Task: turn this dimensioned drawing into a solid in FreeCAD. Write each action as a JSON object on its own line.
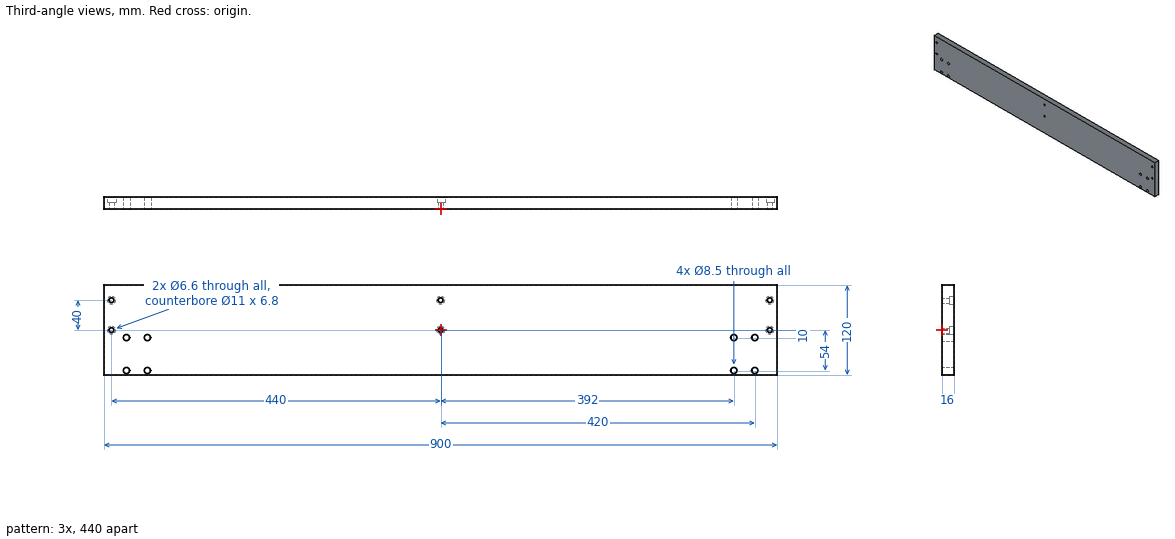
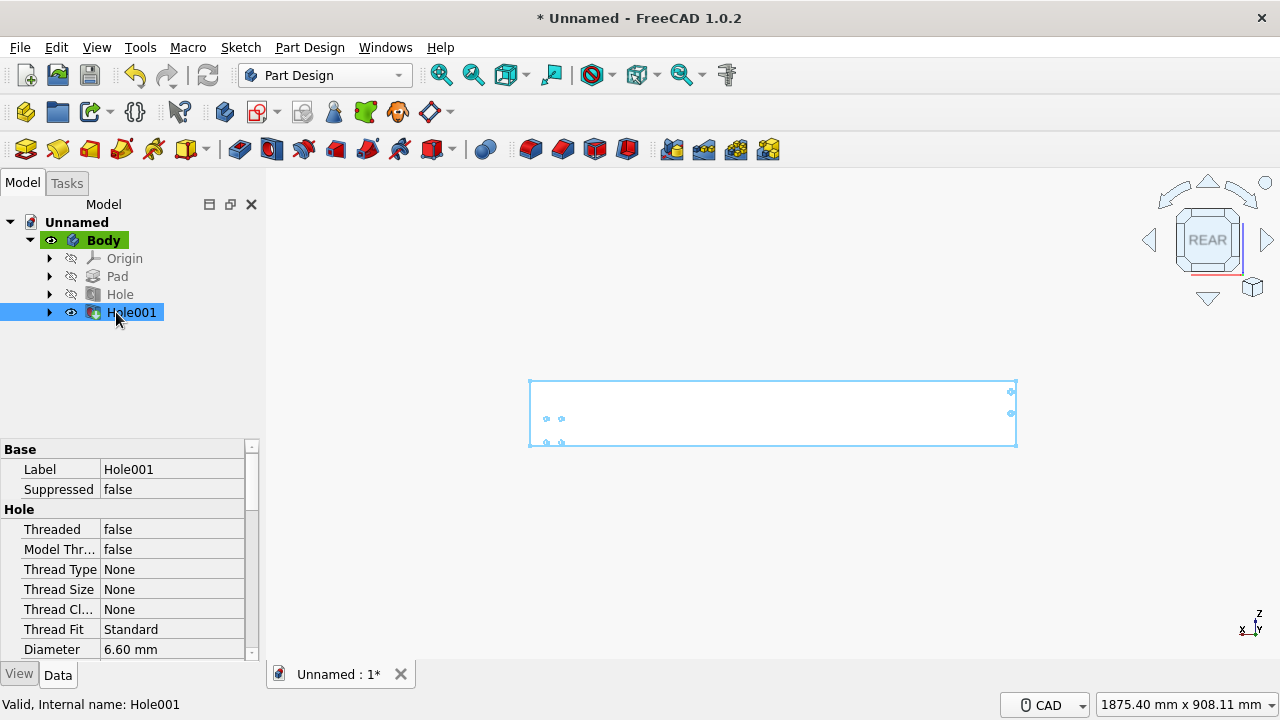
{"action": "left_click", "coordinate": [704, 150]}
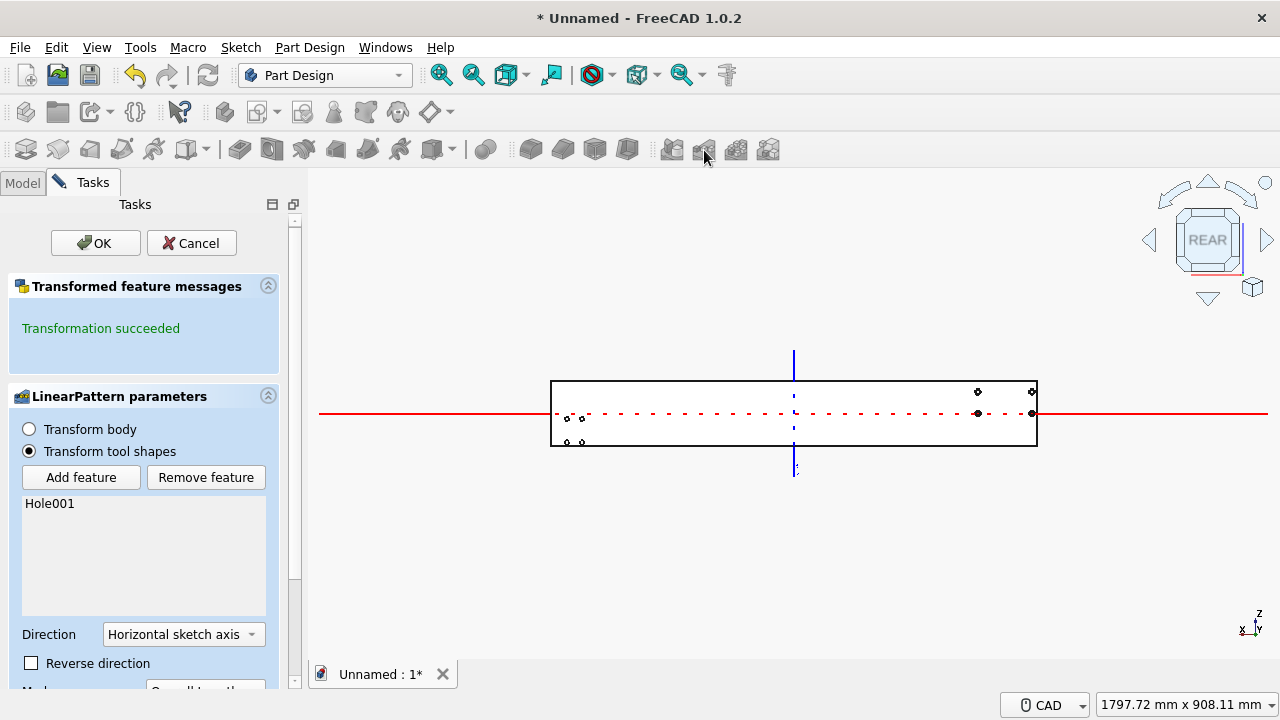
{"action": "left_click", "coordinate": [184, 634]}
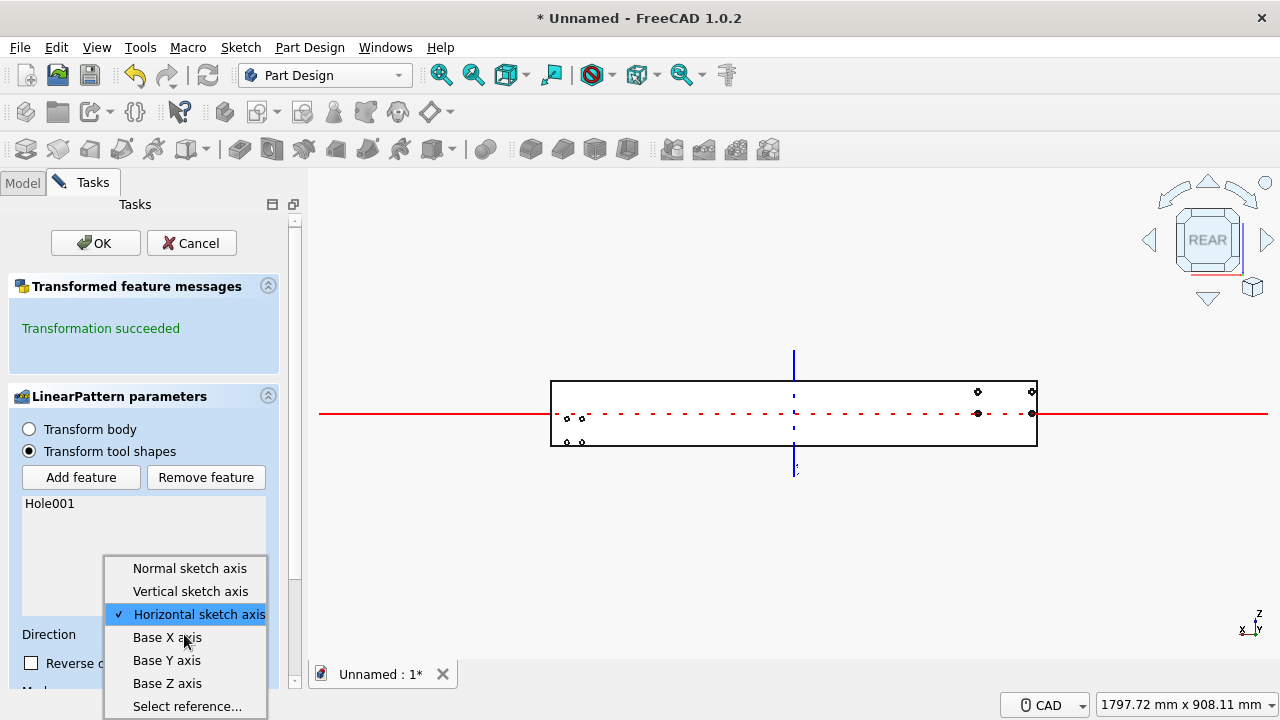
{"action": "left_click", "coordinate": [184, 638]}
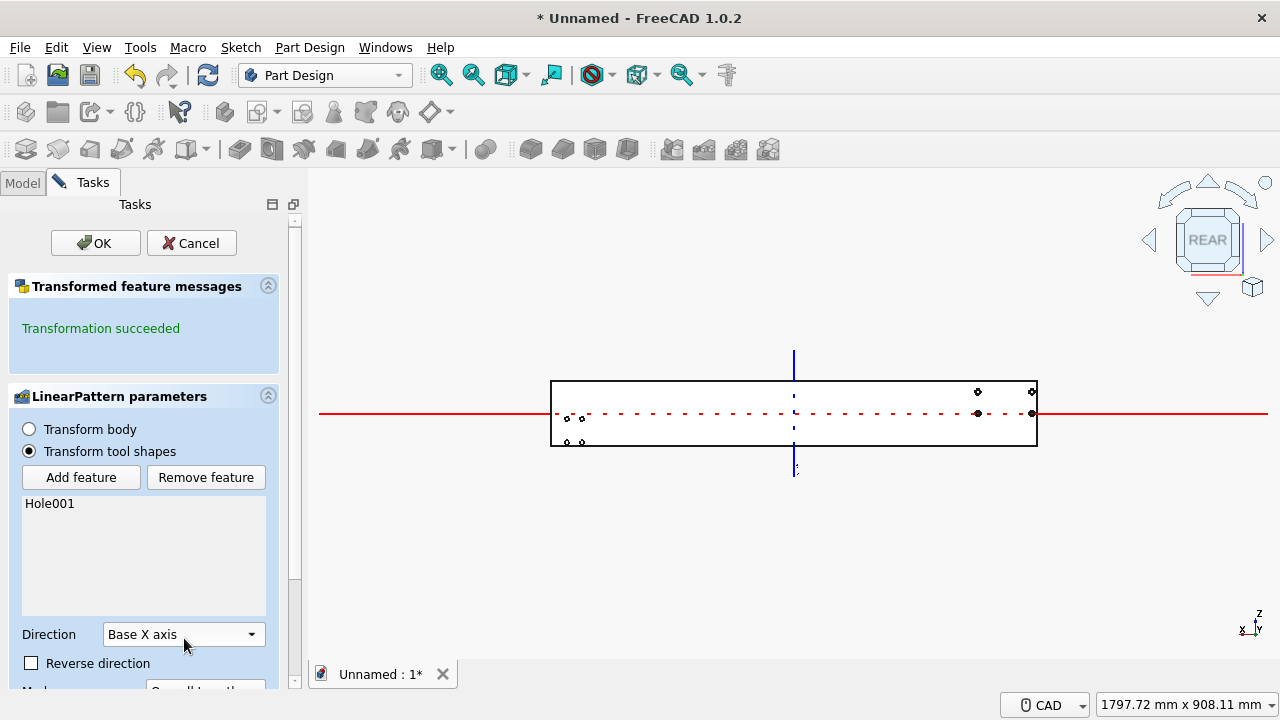
{"action": "scroll", "coordinate": [295, 451], "scroll_direction": "down", "scroll_amount": 2}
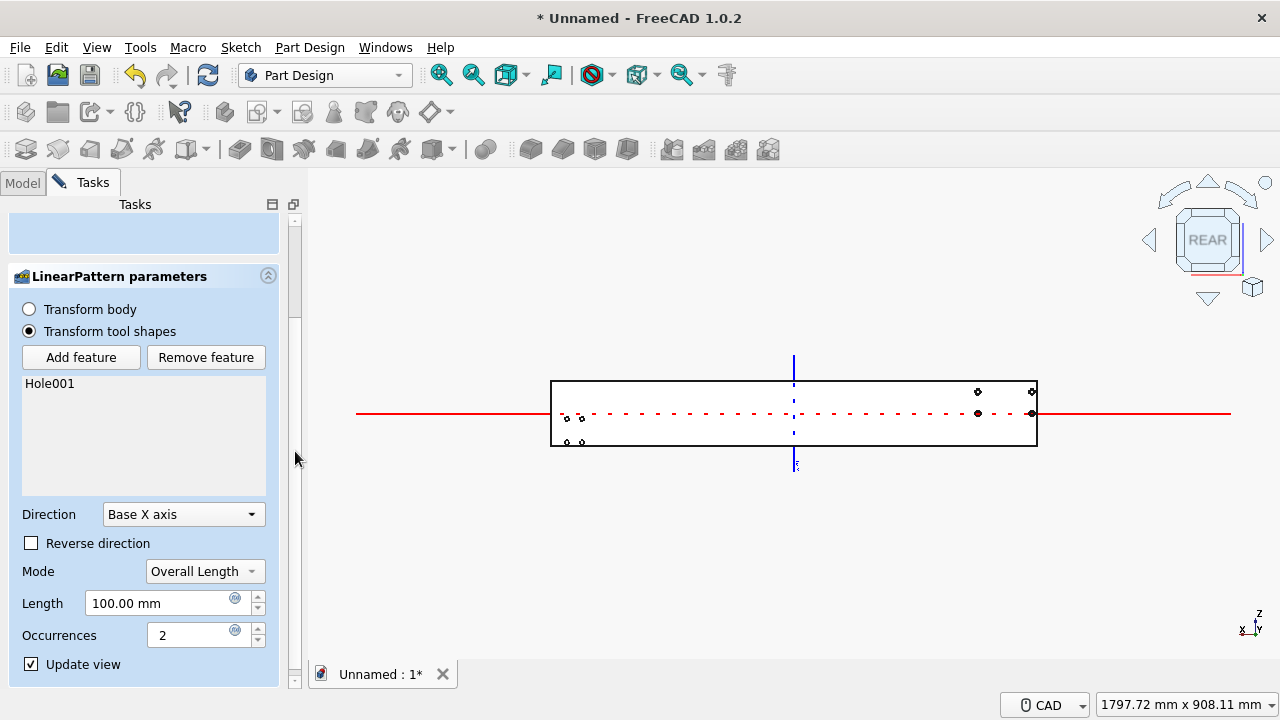
{"action": "left_click", "coordinate": [206, 572]}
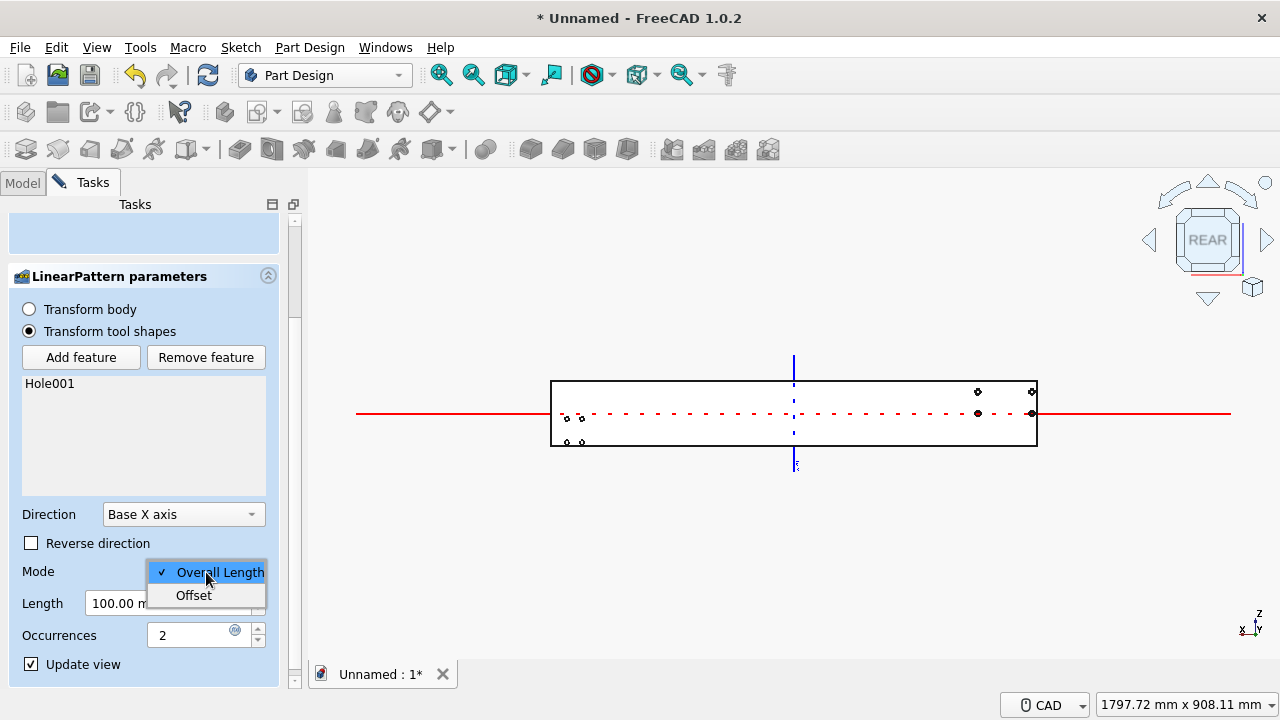
{"action": "left_click", "coordinate": [206, 596]}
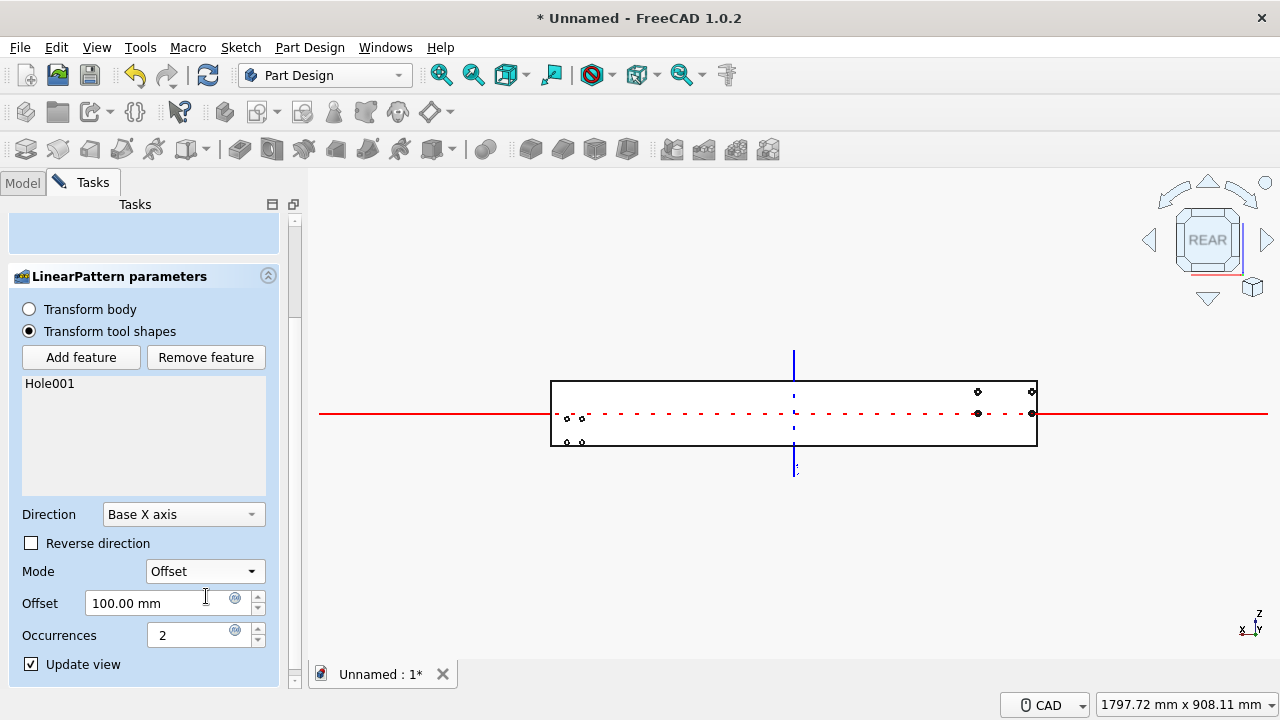
{"action": "triple_click", "coordinate": [168, 603]}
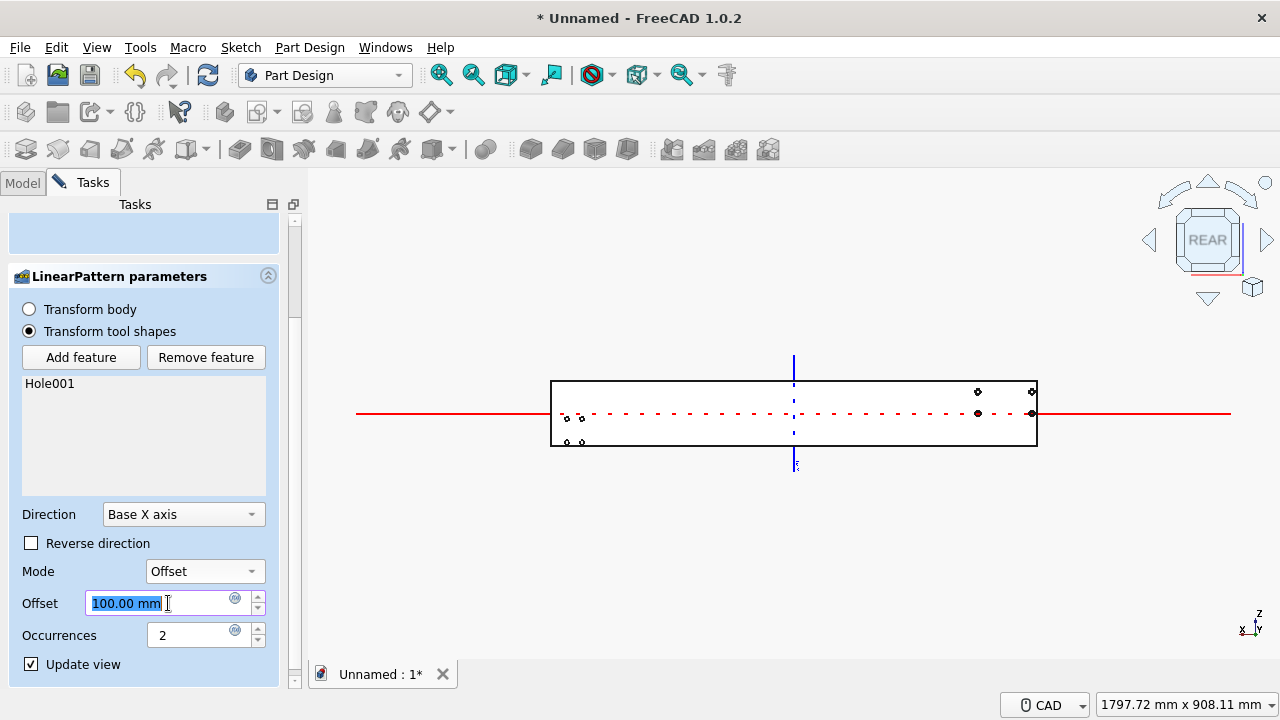
{"action": "type", "text": "440"}
{"action": "key", "text": "Tab"}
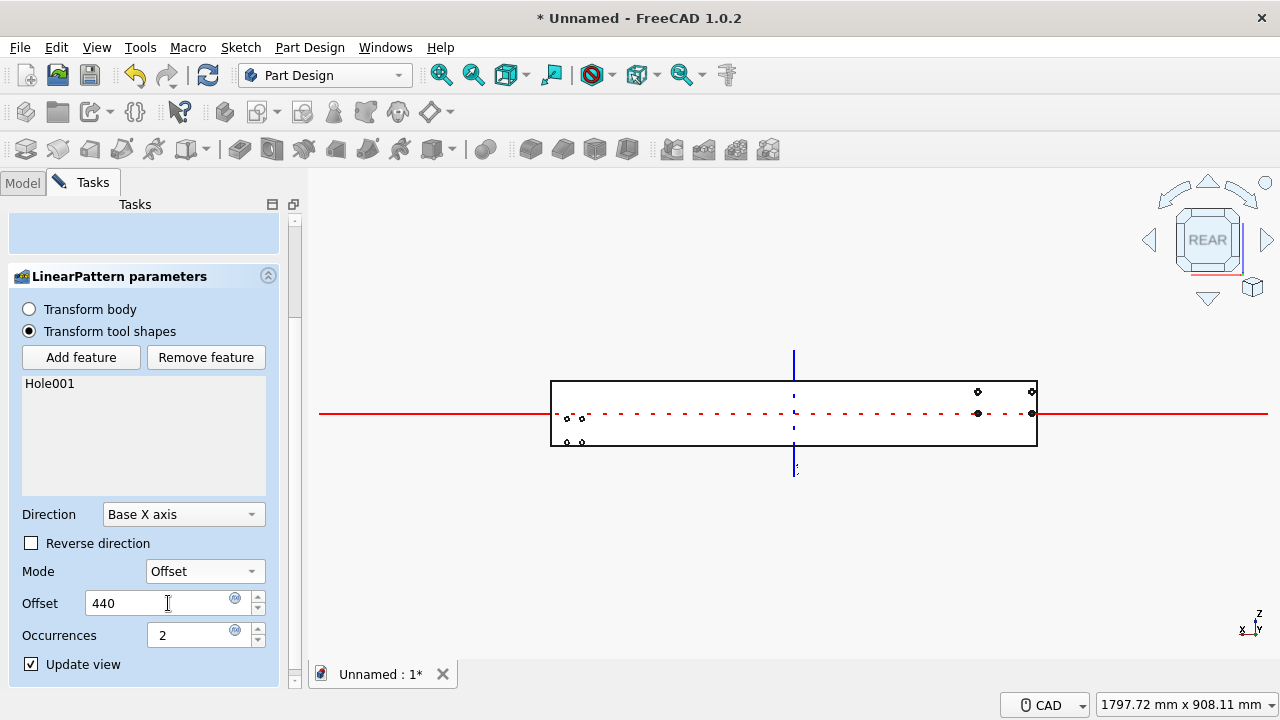
{"action": "triple_click", "coordinate": [198, 635]}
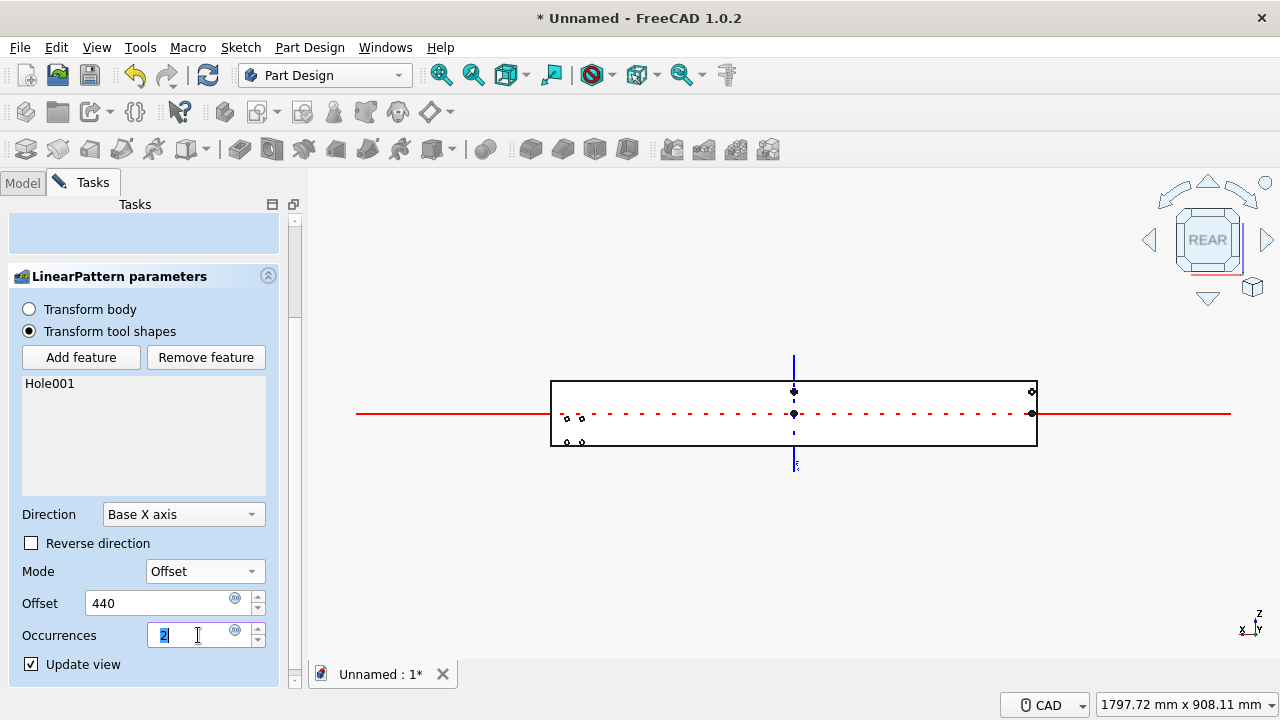
{"action": "type", "text": "3"}
{"action": "key", "text": "Tab"}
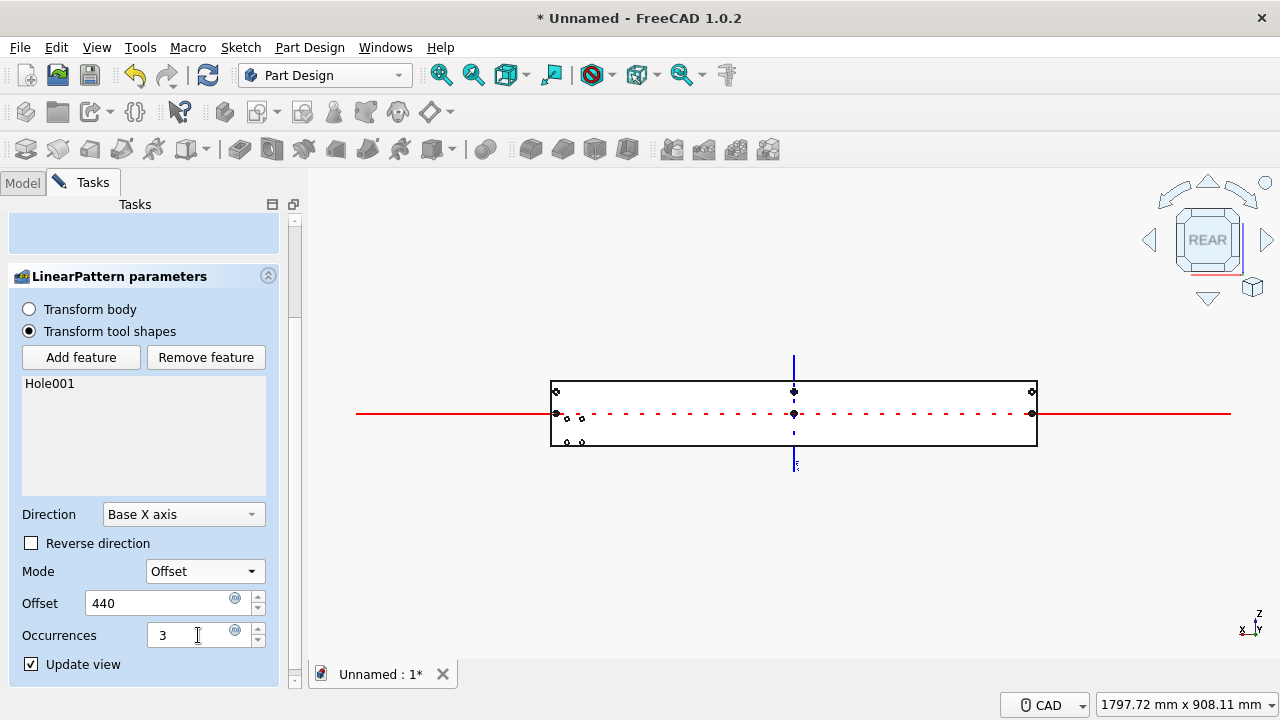
{"action": "scroll", "coordinate": [295, 451], "scroll_direction": "up", "scroll_amount": 3}